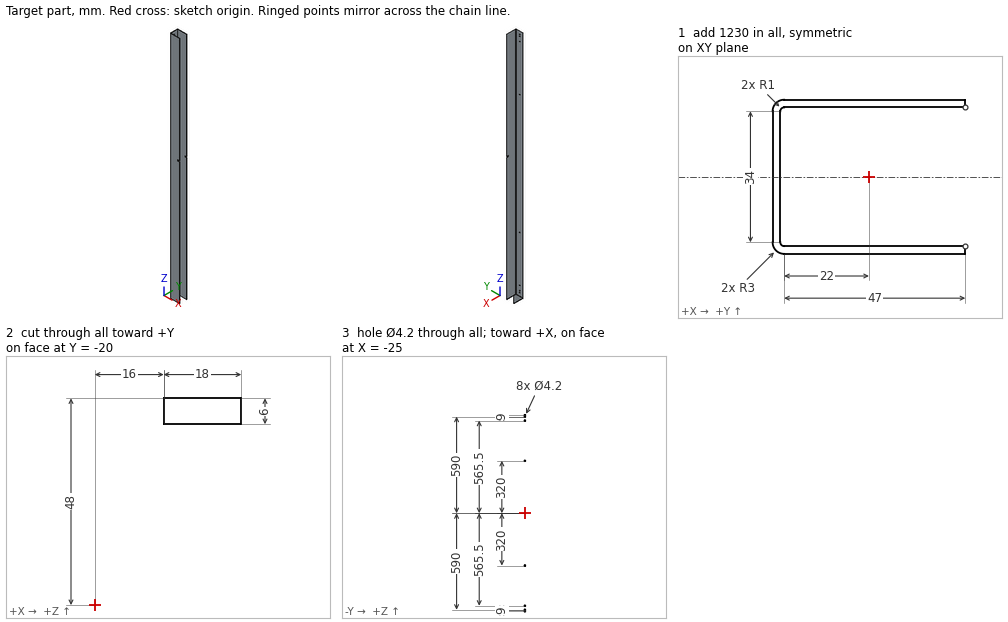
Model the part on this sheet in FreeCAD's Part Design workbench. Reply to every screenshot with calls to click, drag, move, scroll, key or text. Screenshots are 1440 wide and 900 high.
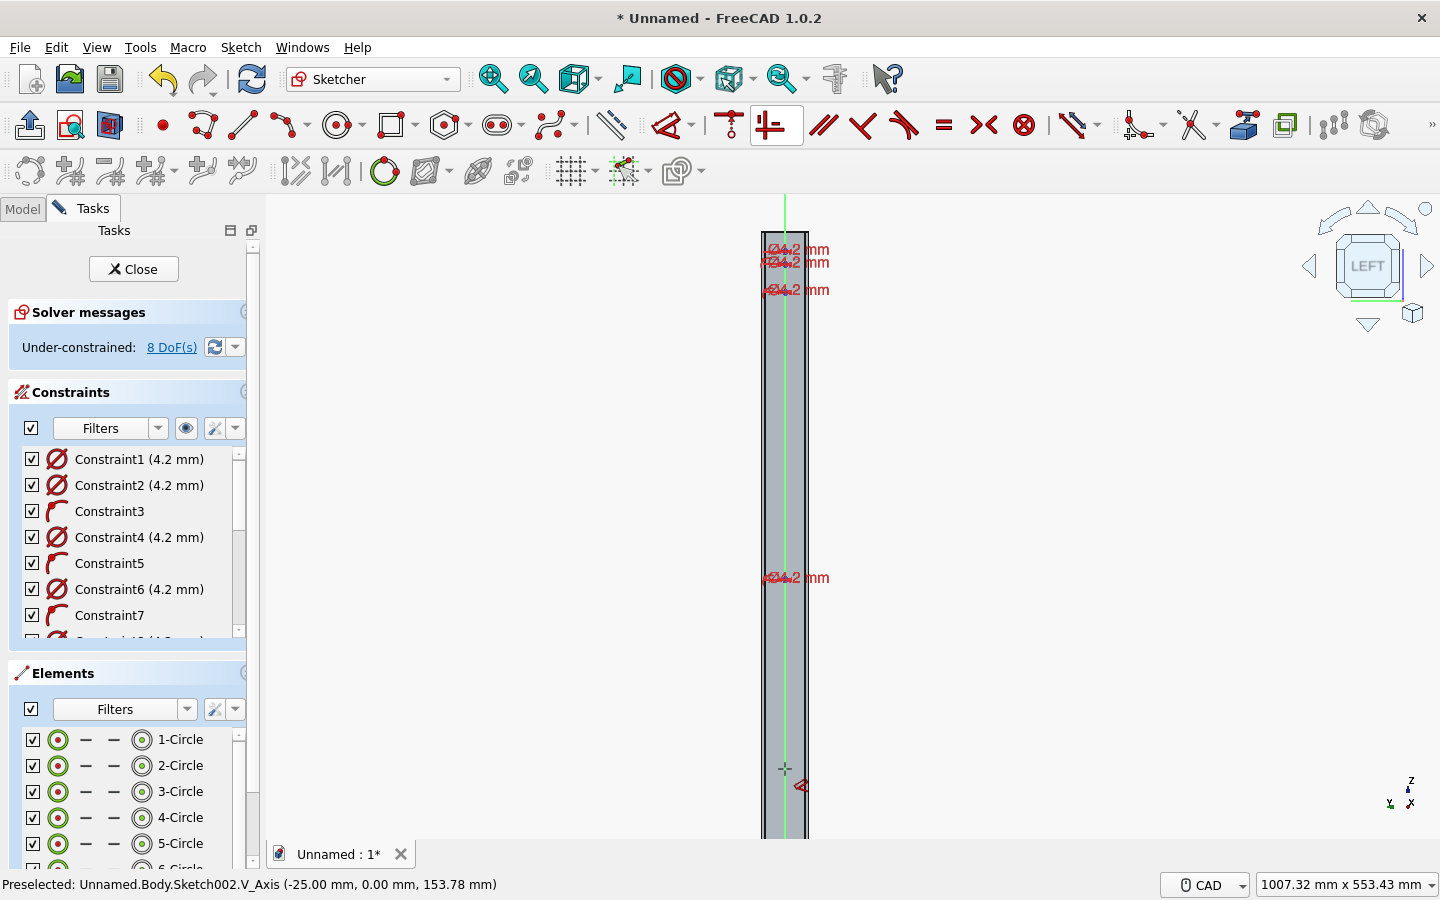
scroll(785, 264, up, 7)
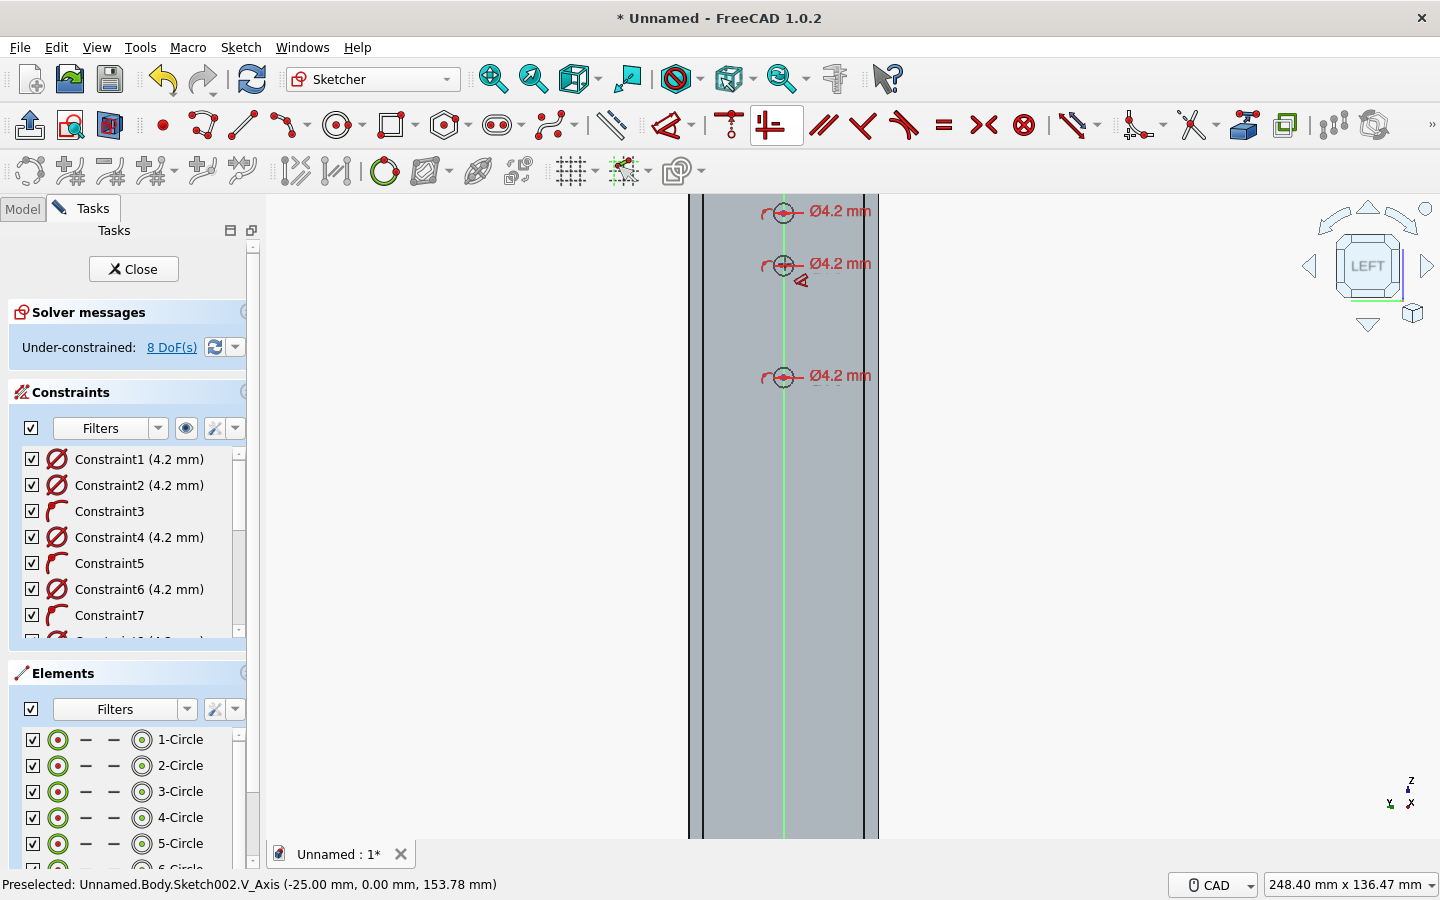
click(784, 266)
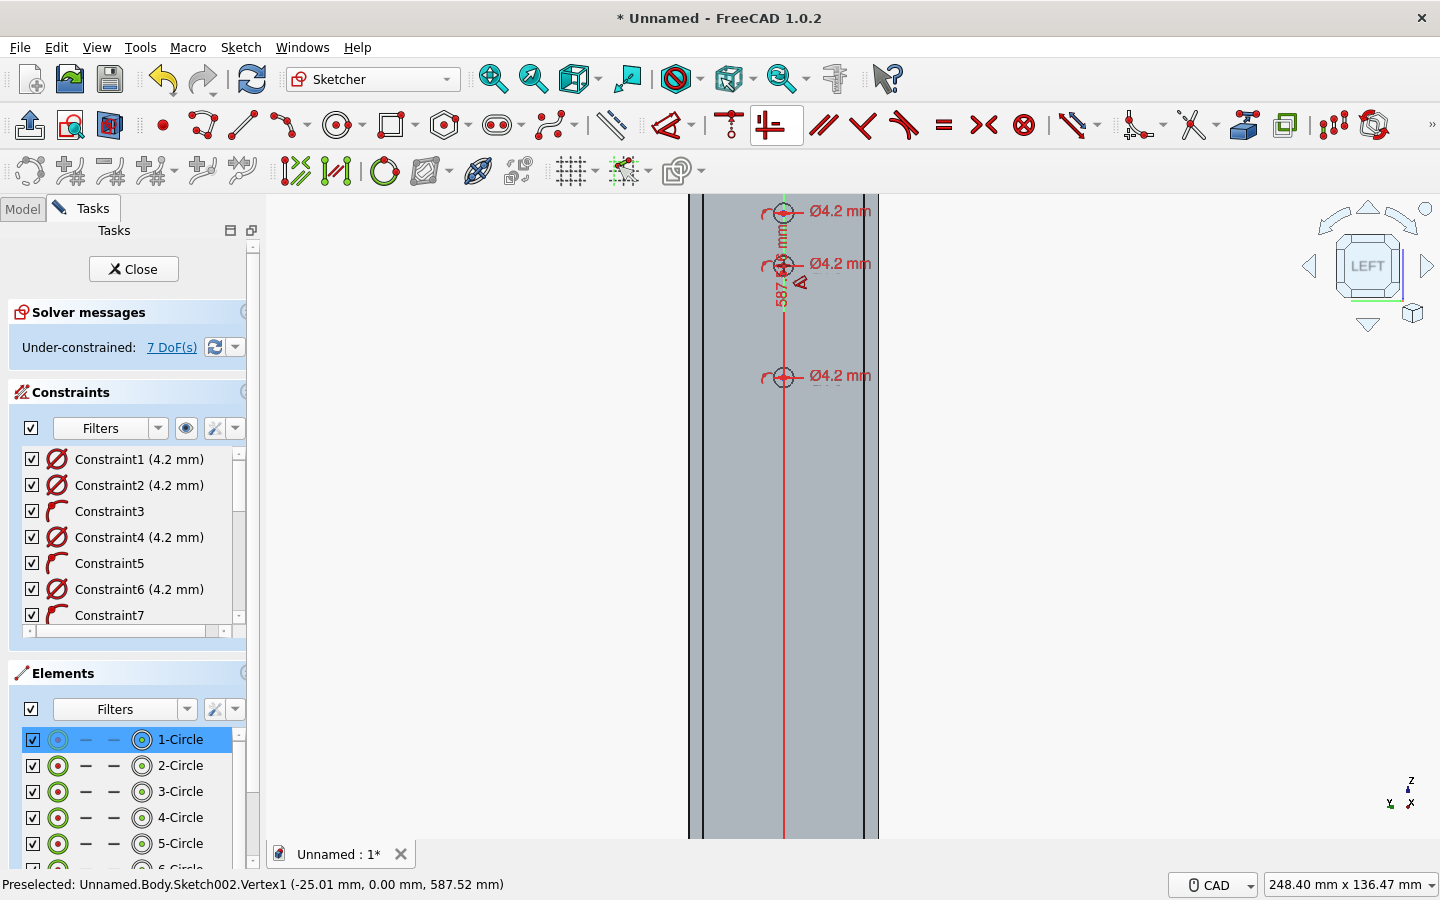
scroll(785, 314, down, 13)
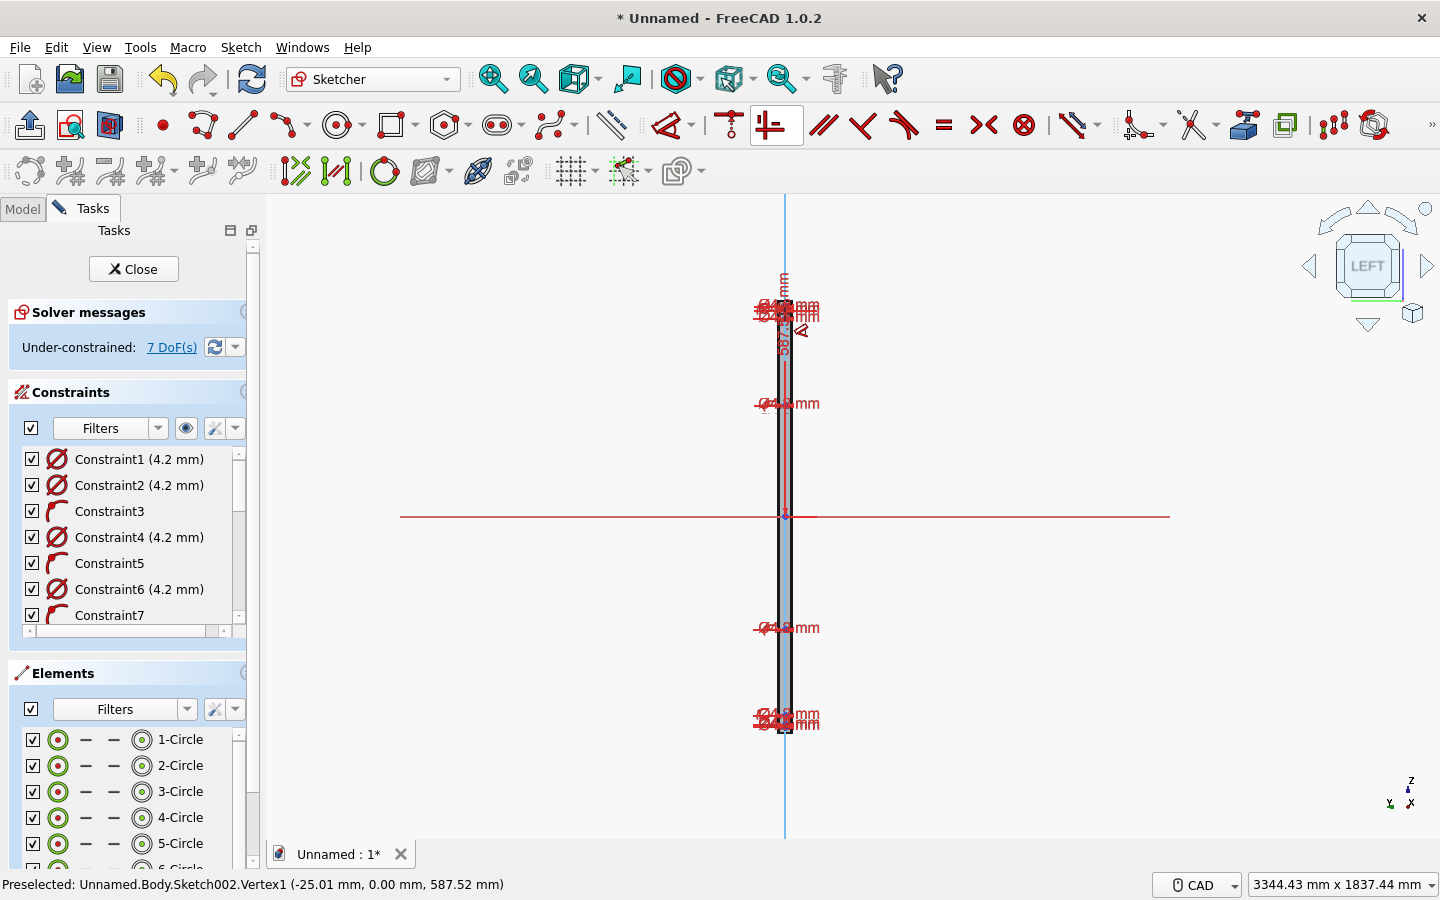
scroll(785, 307, up, 13)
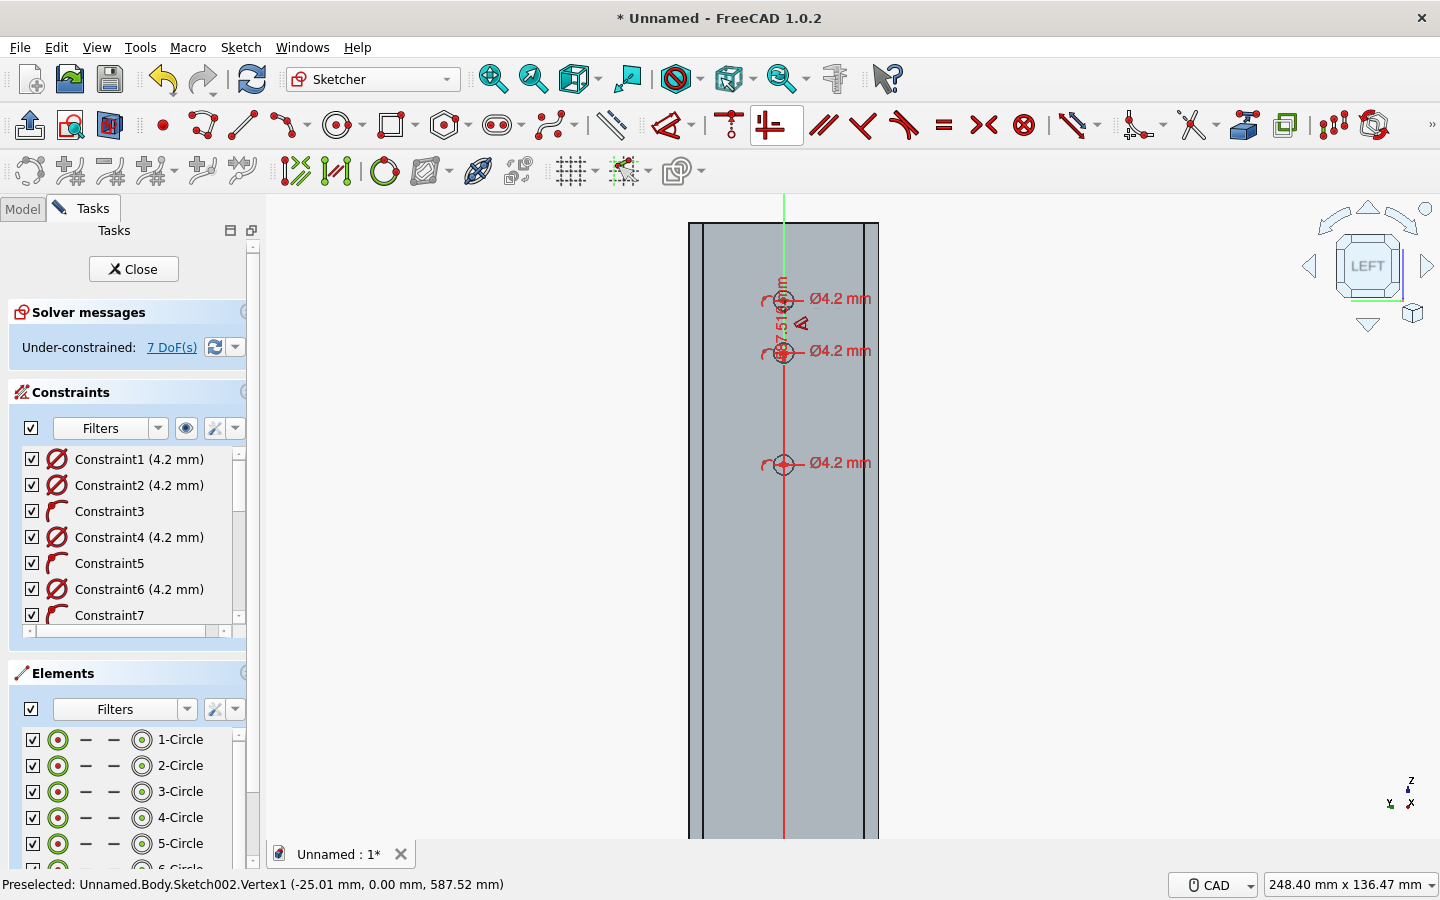
click(784, 301)
click(818, 327)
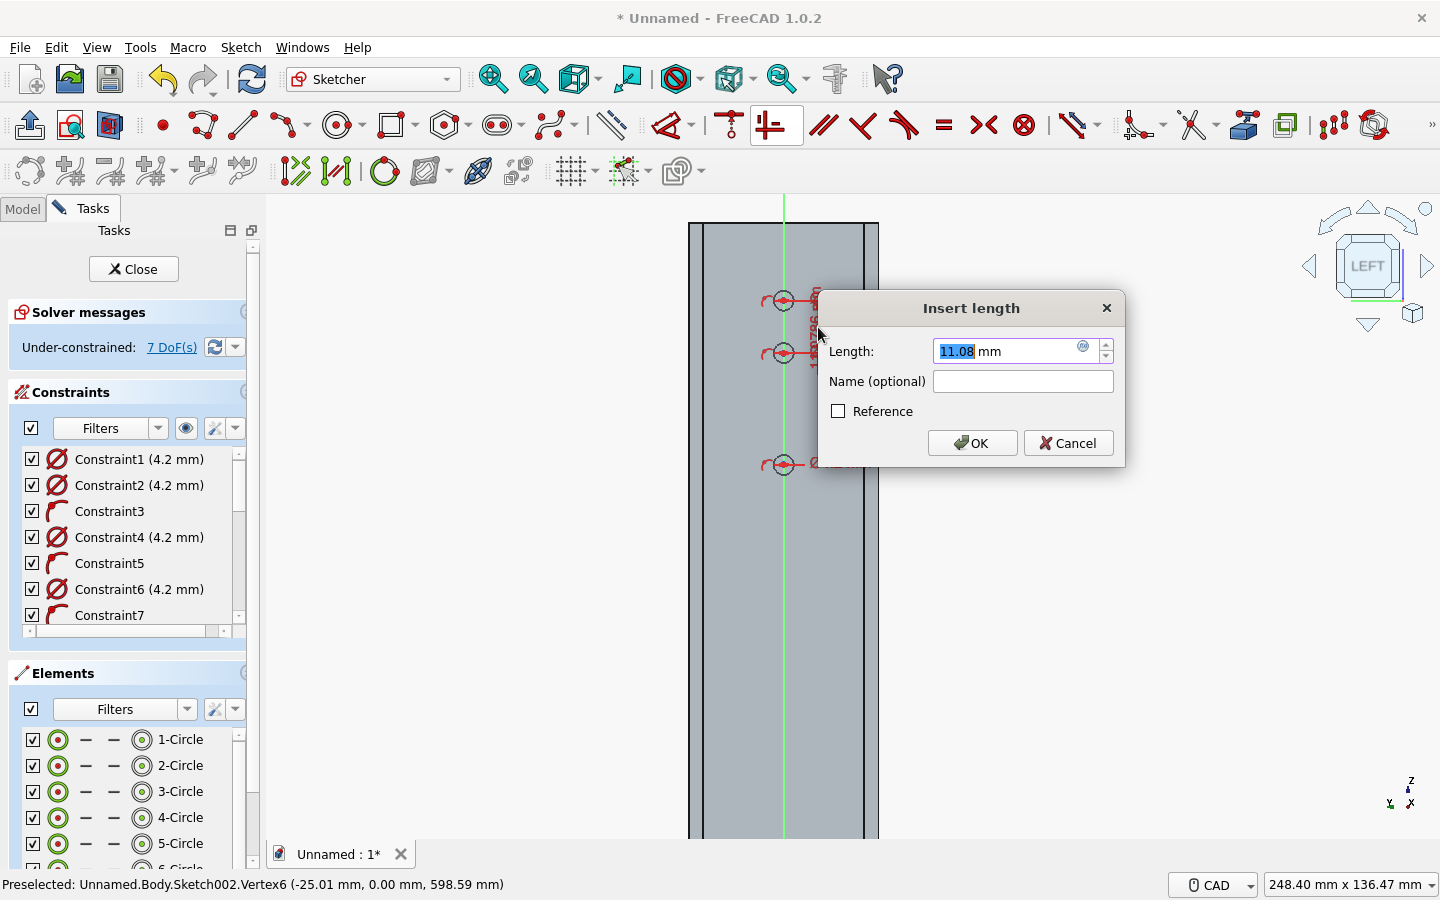
text(9)
key(Return)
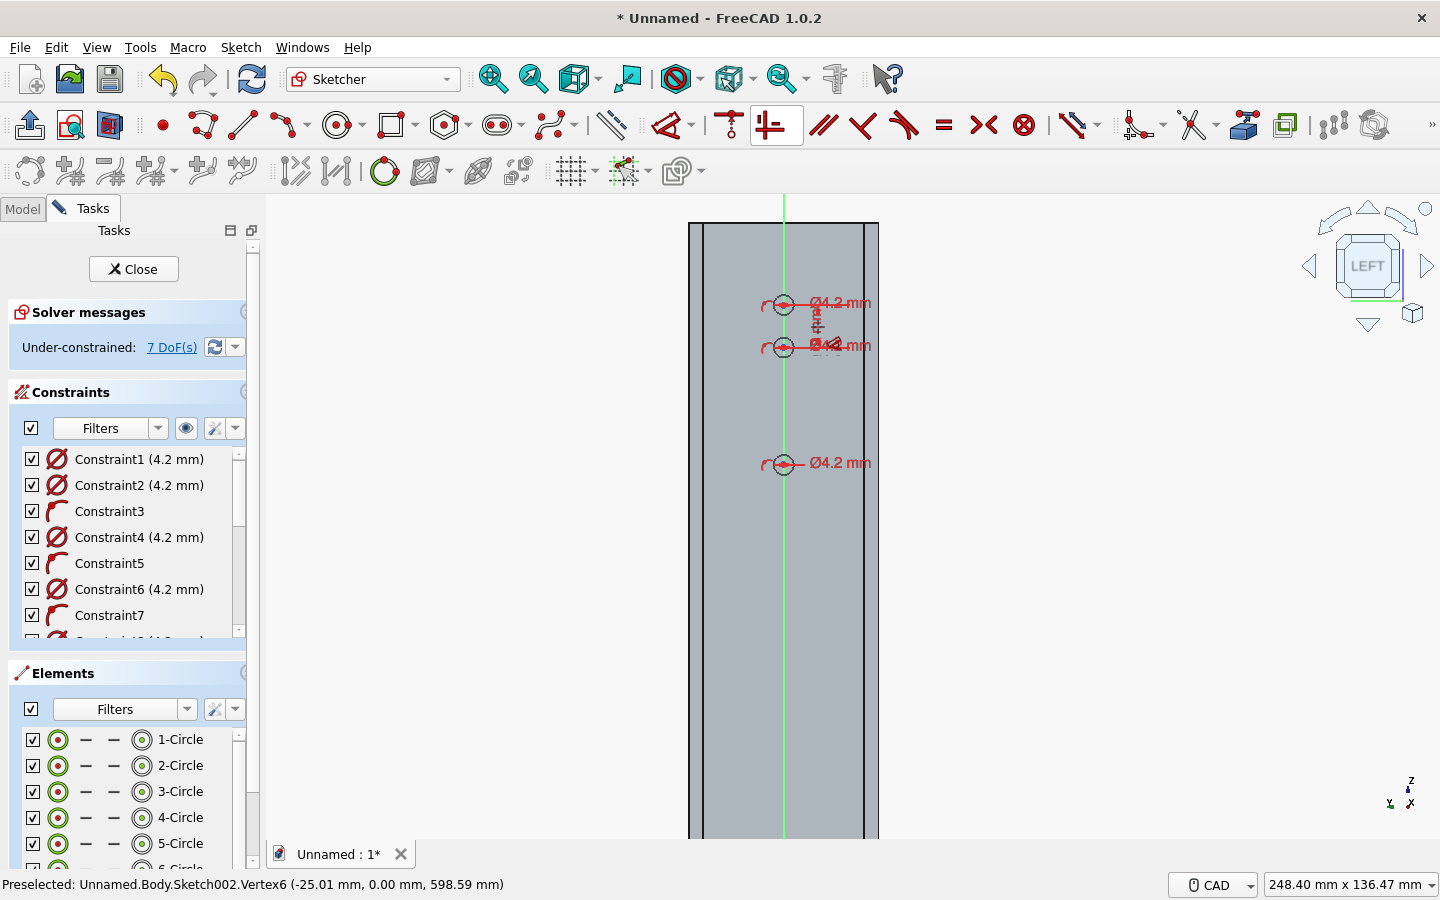
scroll(785, 307, down, 13)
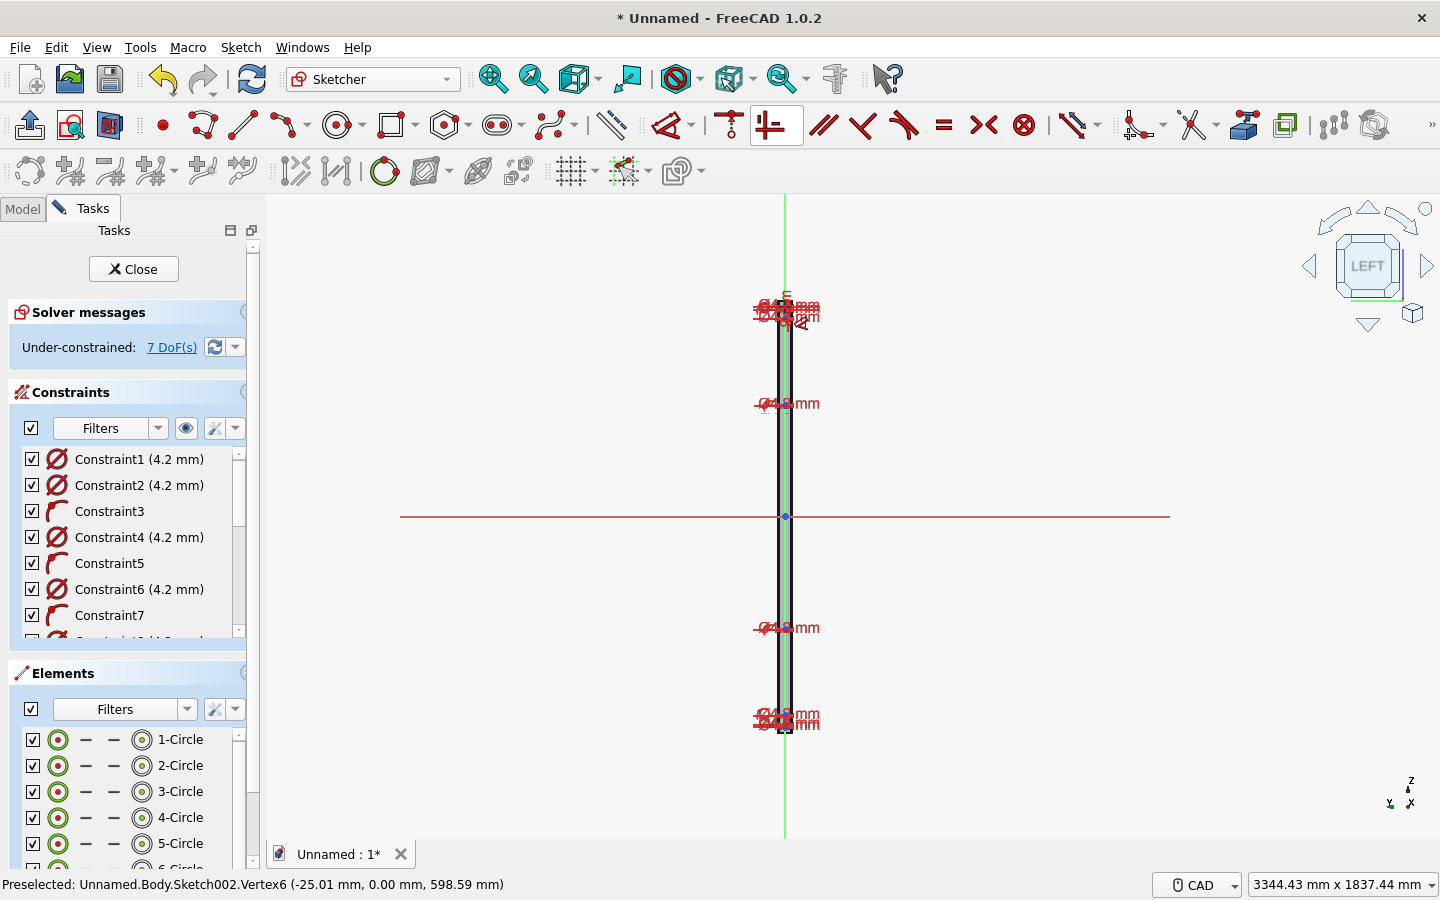
scroll(785, 725, up, 13)